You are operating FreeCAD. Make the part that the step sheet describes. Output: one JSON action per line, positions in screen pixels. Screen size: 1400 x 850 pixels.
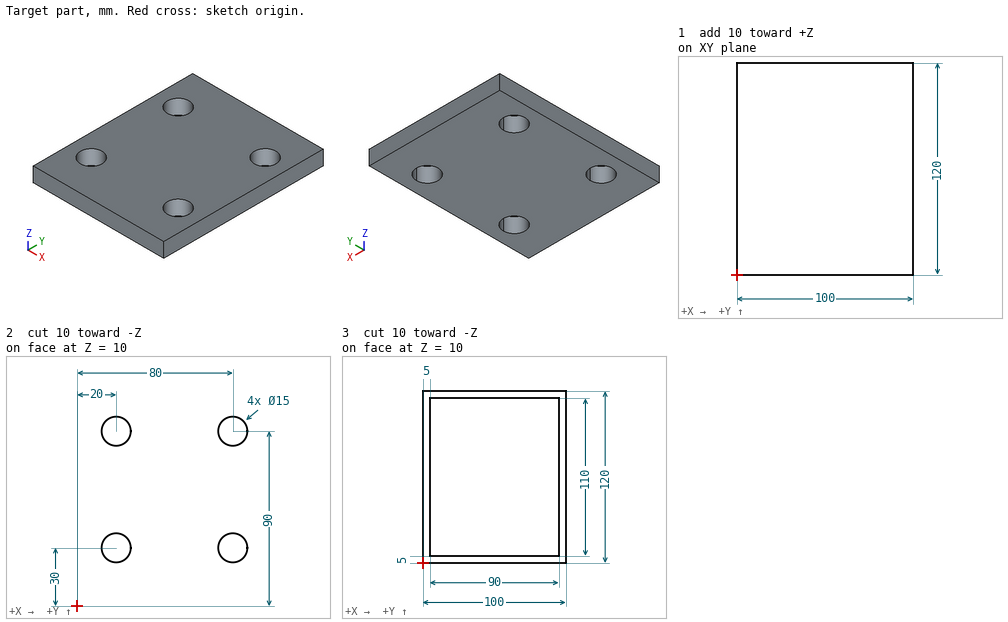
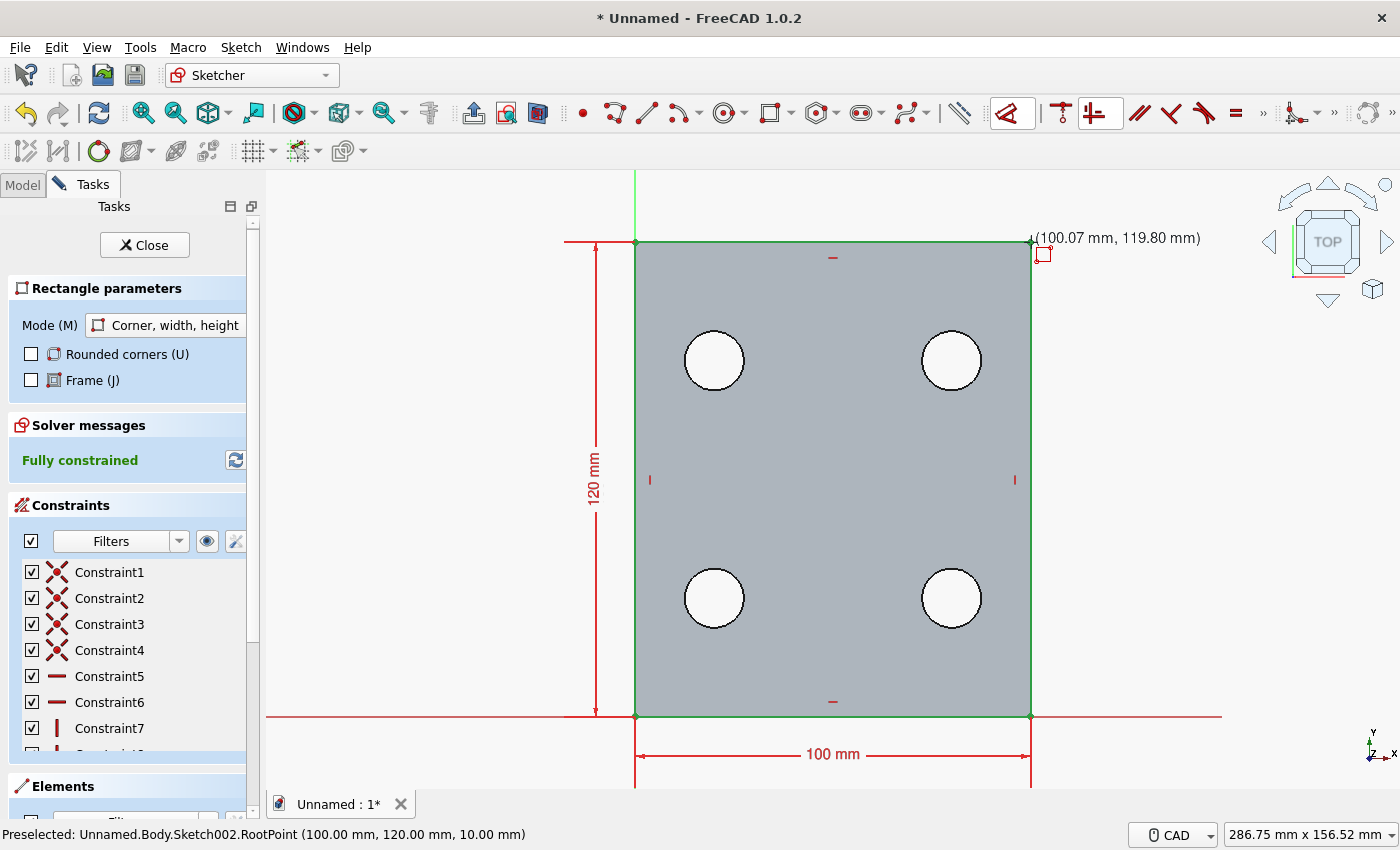
{"action": "left_click", "coordinate": [655, 262]}
{"action": "mouse_move", "coordinate": [1011, 697]}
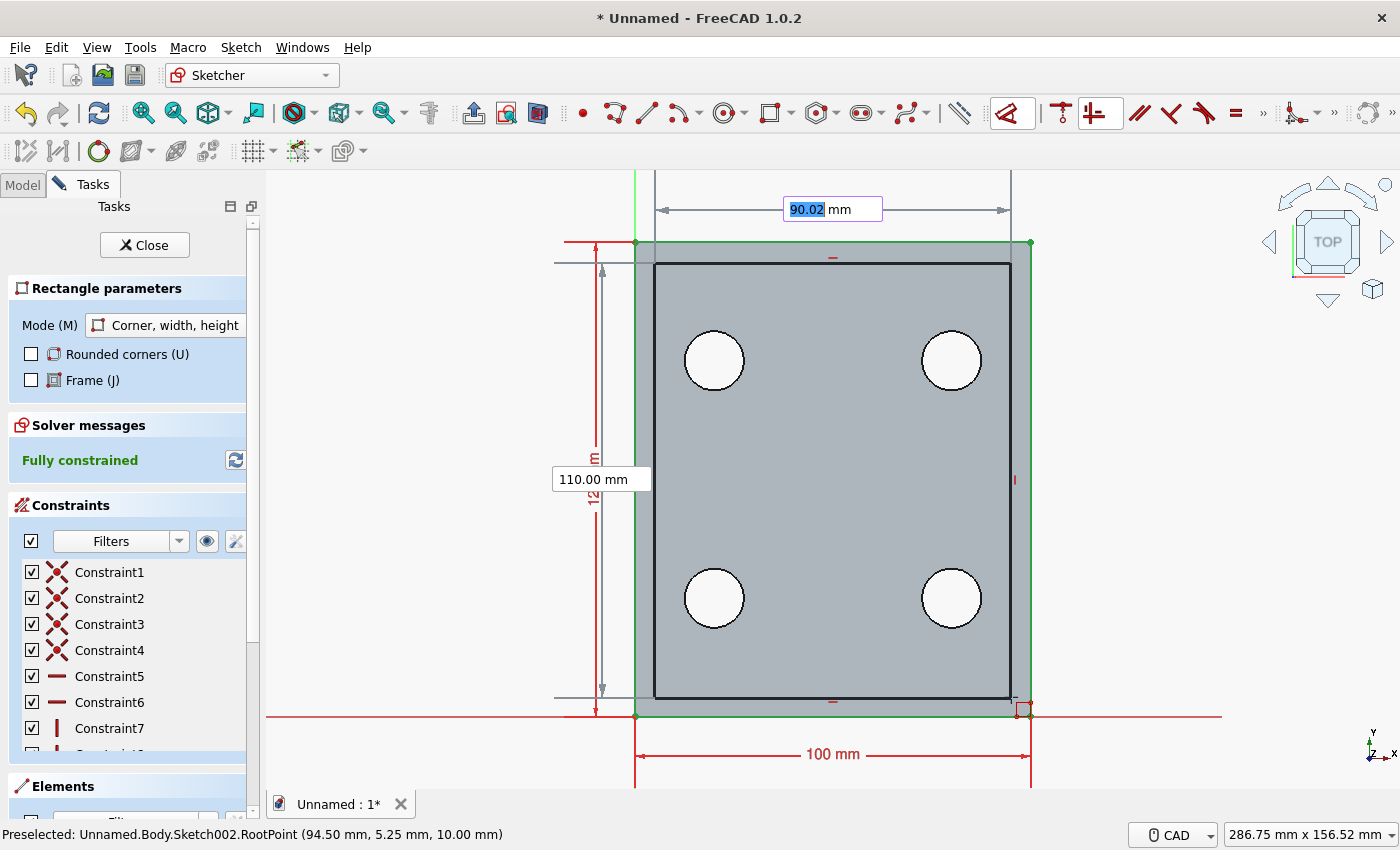
{"action": "type", "text": "90"}
{"action": "key", "text": "Tab"}
{"action": "type", "text": "110"}
{"action": "key", "text": "Return"}
{"action": "key", "text": "Escape"}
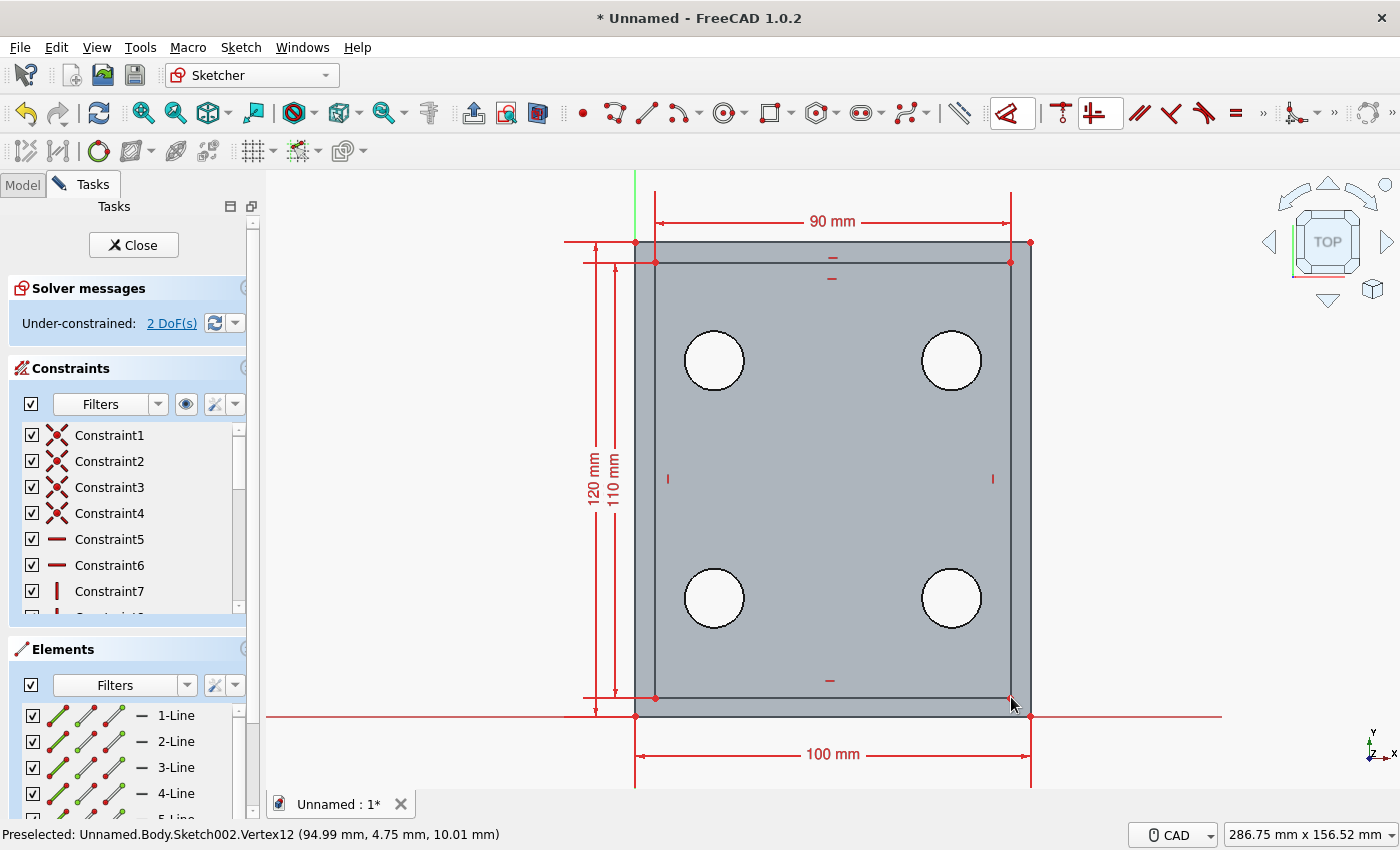
{"action": "key", "text": "d"}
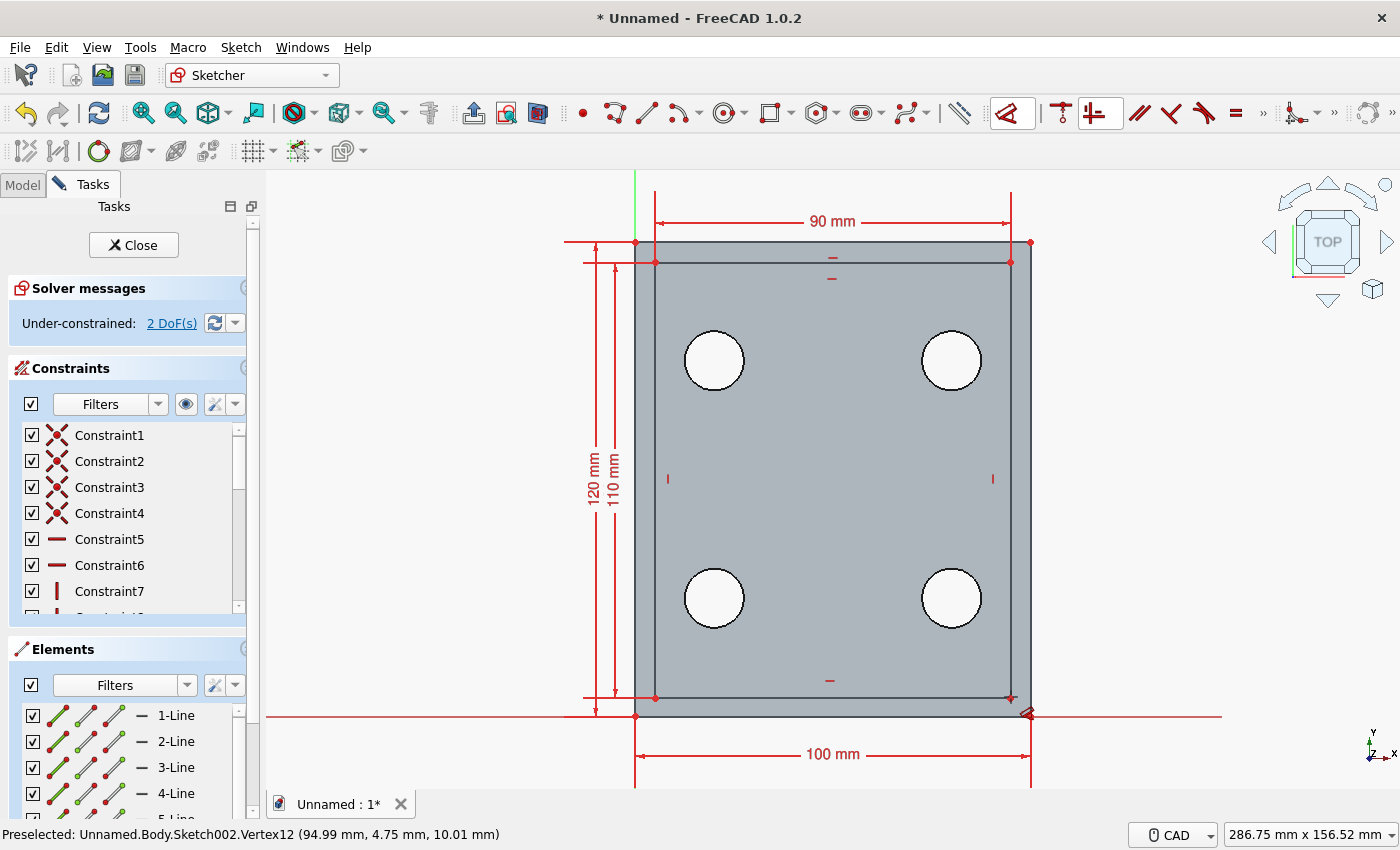
{"action": "scroll", "coordinate": [655, 263], "scroll_direction": "up", "scroll_amount": 4}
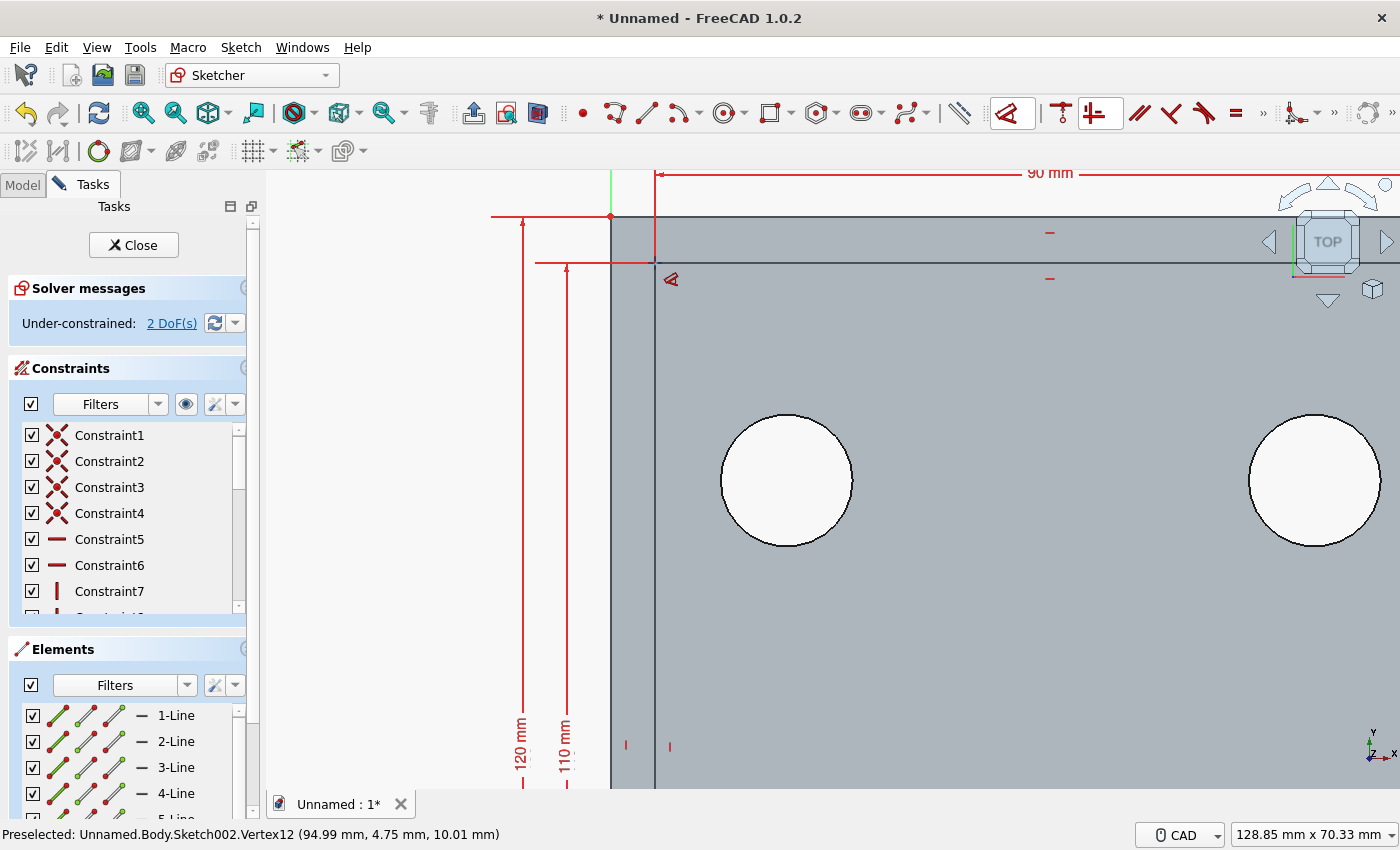
{"action": "left_click", "coordinate": [655, 263]}
{"action": "left_click", "coordinate": [633, 229]}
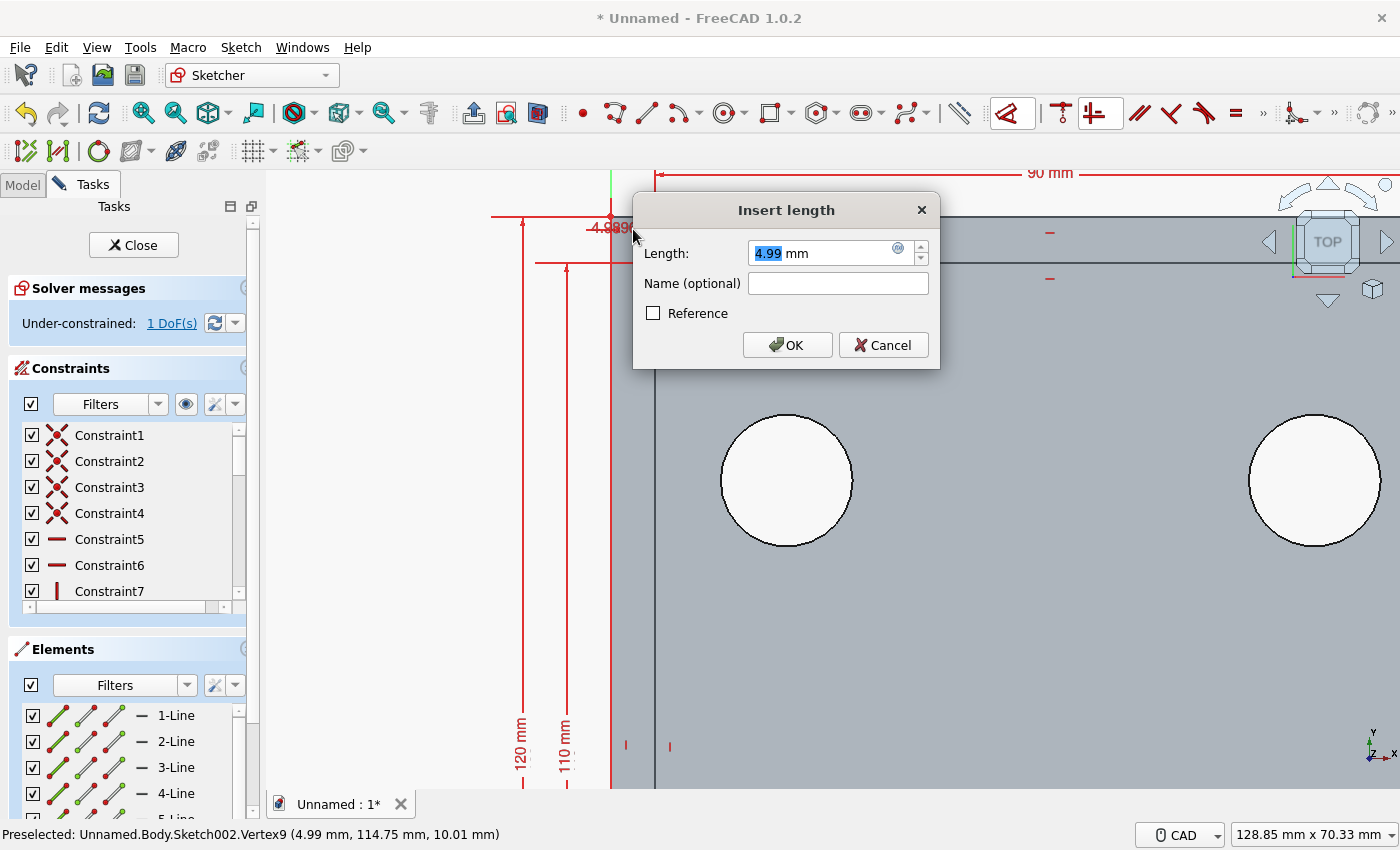
{"action": "type", "text": "5"}
{"action": "key", "text": "Return"}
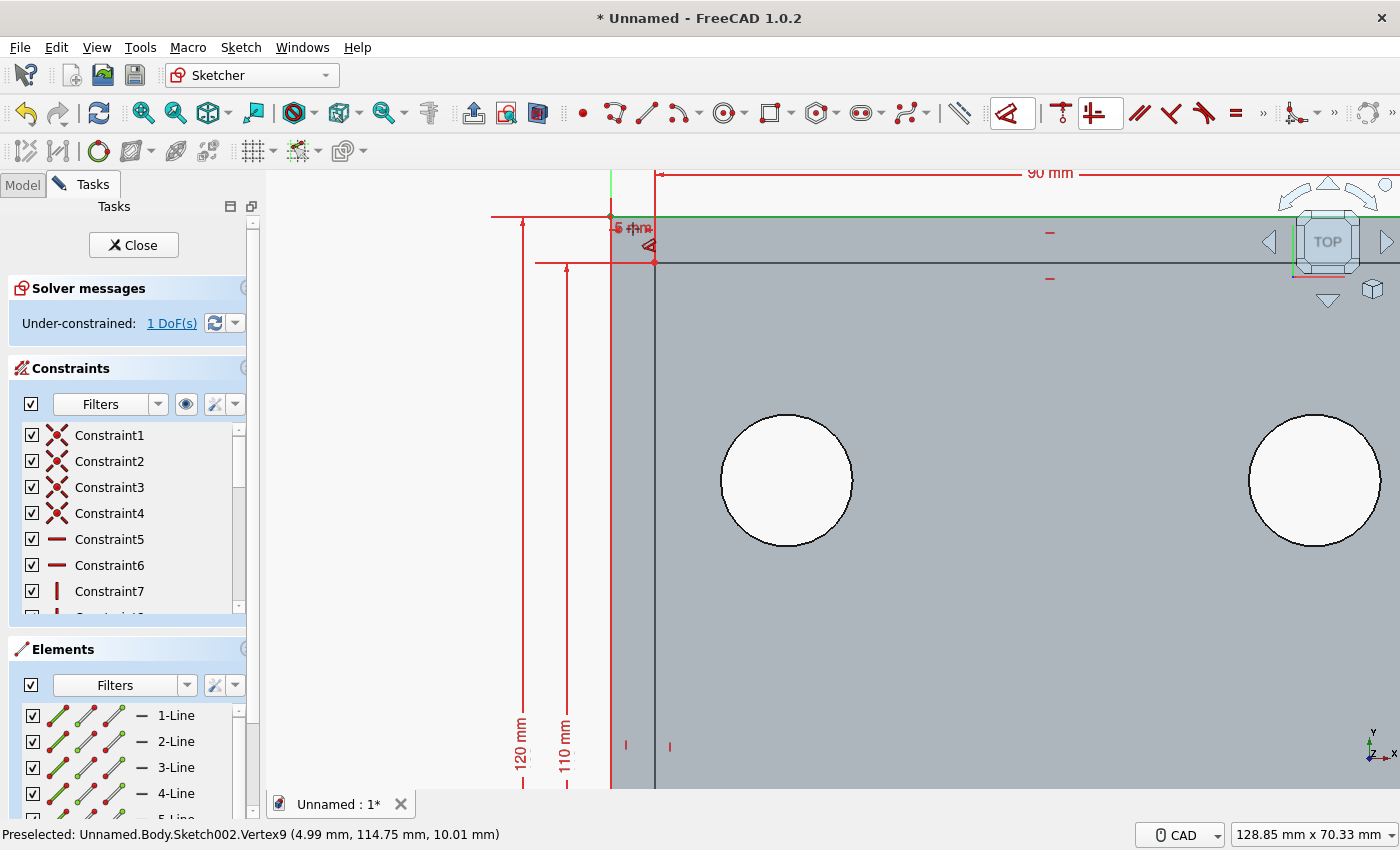
{"action": "scroll", "coordinate": [598, 325], "scroll_direction": "down", "scroll_amount": 5}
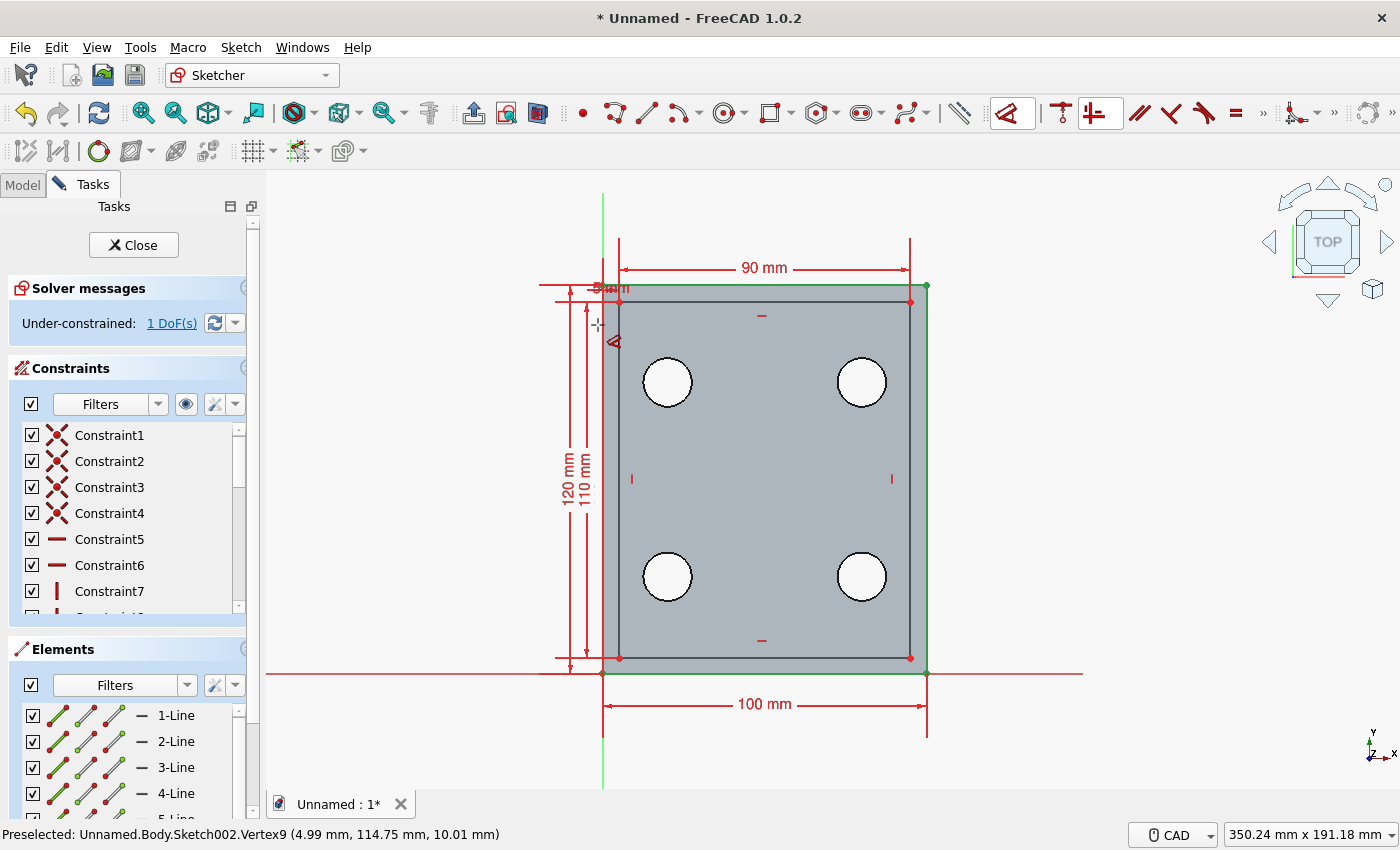
{"action": "scroll", "coordinate": [619, 658], "scroll_direction": "up", "scroll_amount": 5}